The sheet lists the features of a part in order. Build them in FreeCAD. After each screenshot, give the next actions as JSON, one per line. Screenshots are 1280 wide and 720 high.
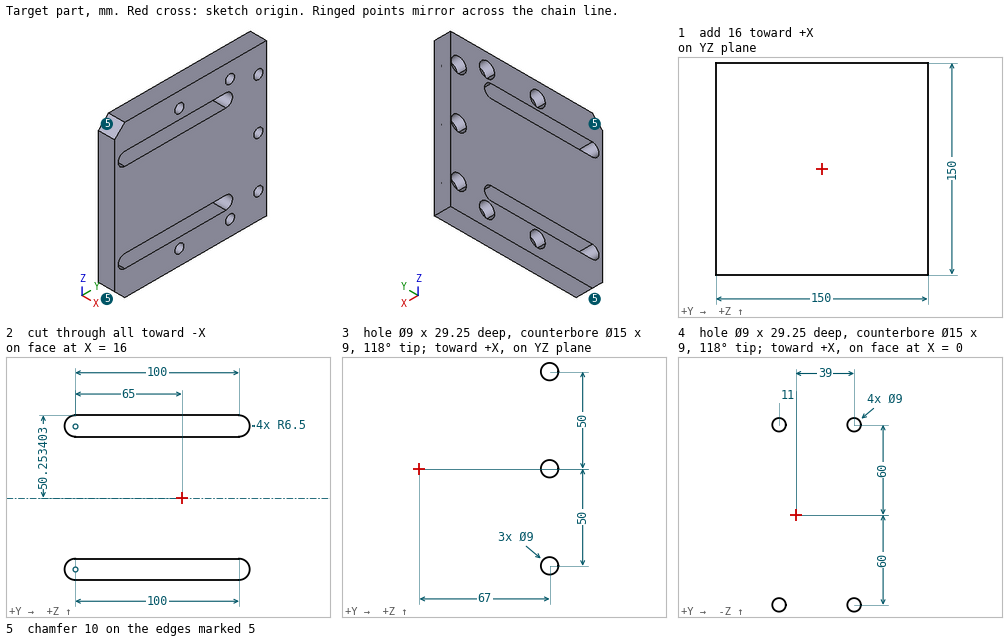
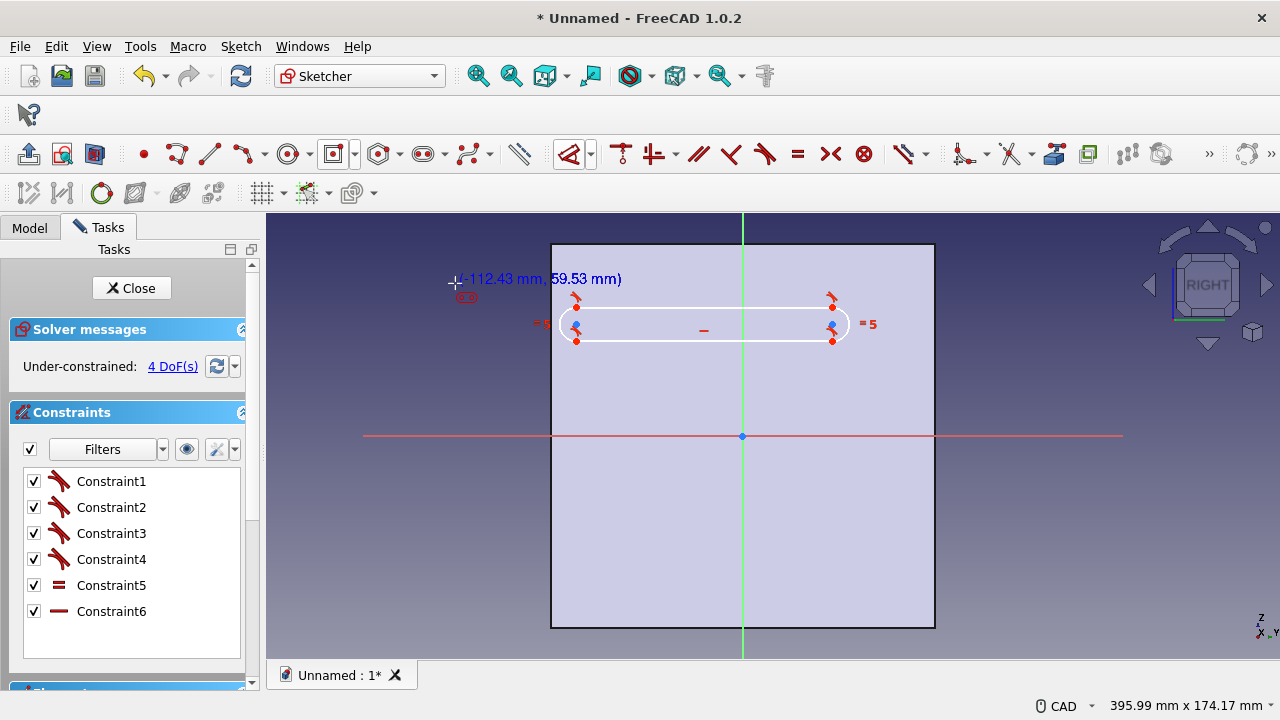
{"action": "scroll", "coordinate": [577, 548], "scroll_direction": "up", "scroll_amount": 2}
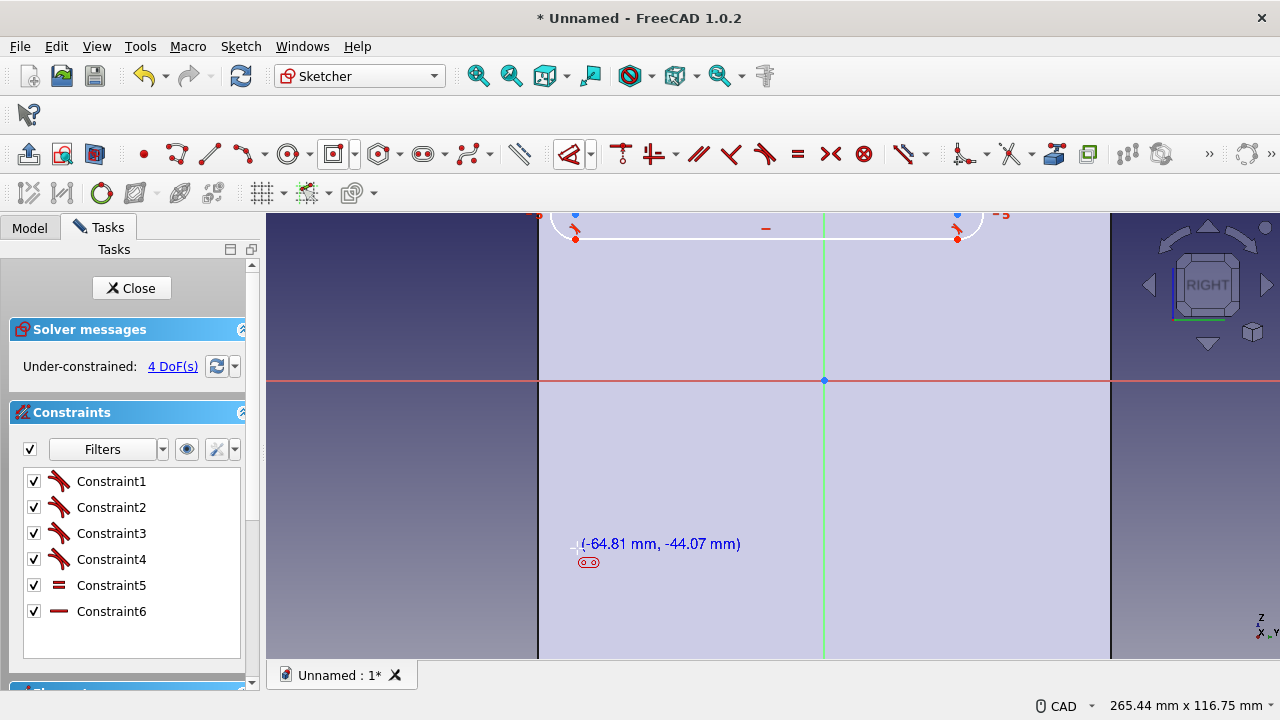
{"action": "left_click", "coordinate": [576, 548]}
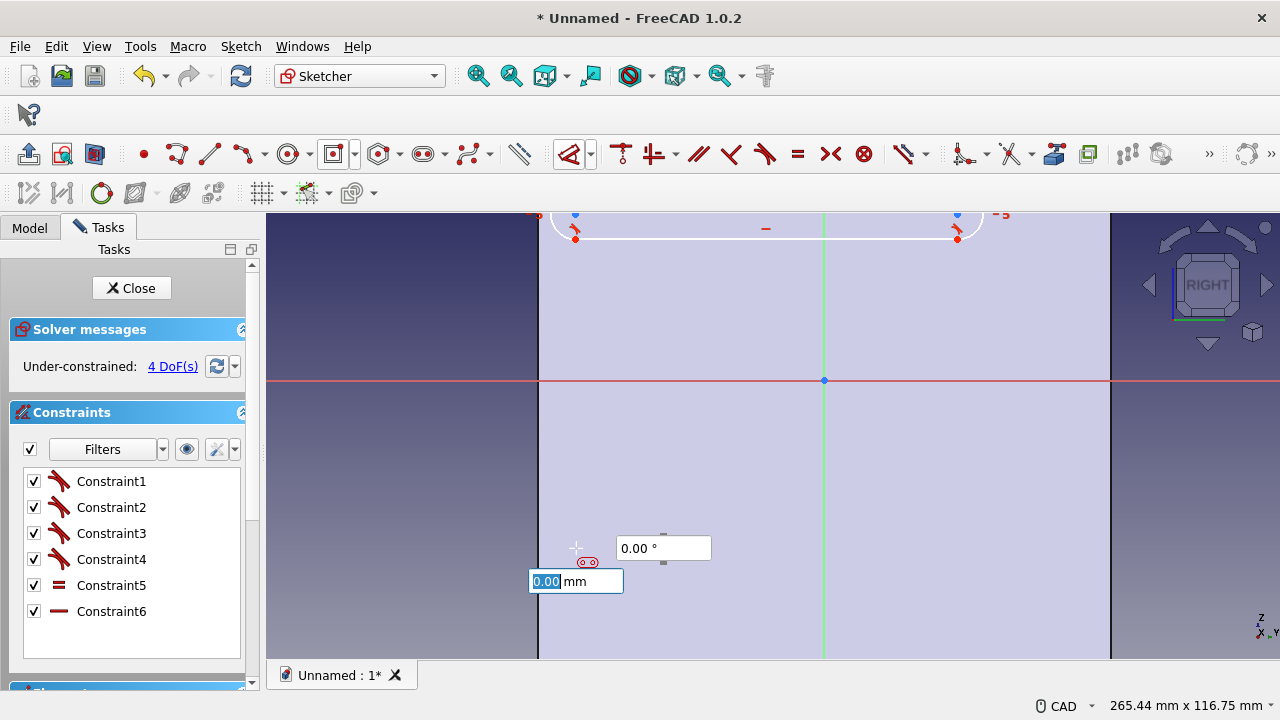
{"action": "left_click", "coordinate": [958, 548]}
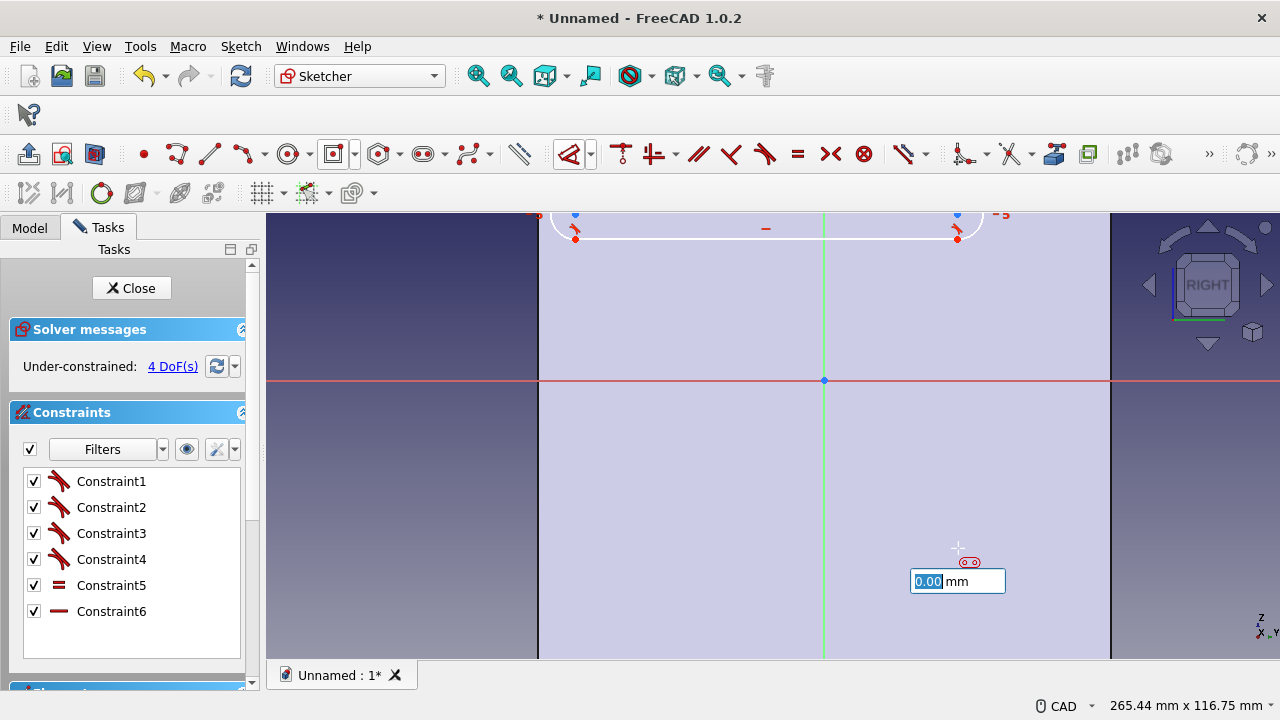
{"action": "left_click", "coordinate": [767, 573]}
{"action": "key", "text": "Escape"}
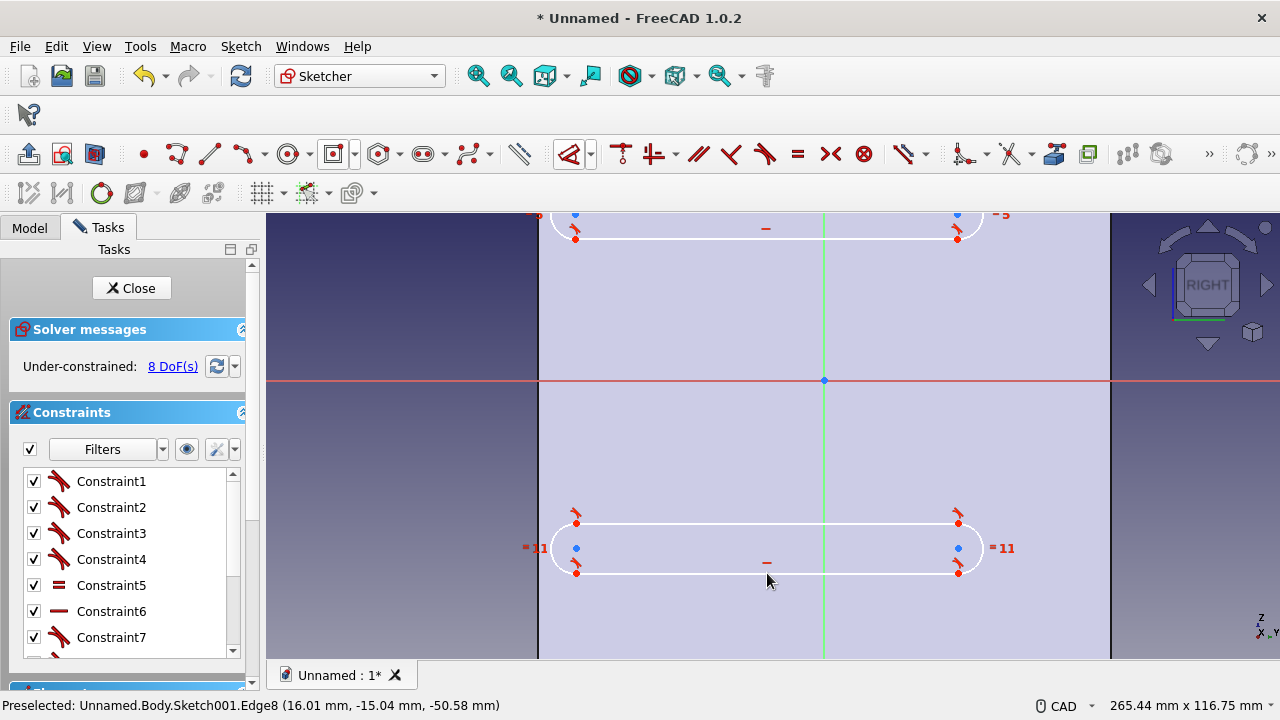
{"action": "scroll", "coordinate": [577, 548], "scroll_direction": "down", "scroll_amount": 2}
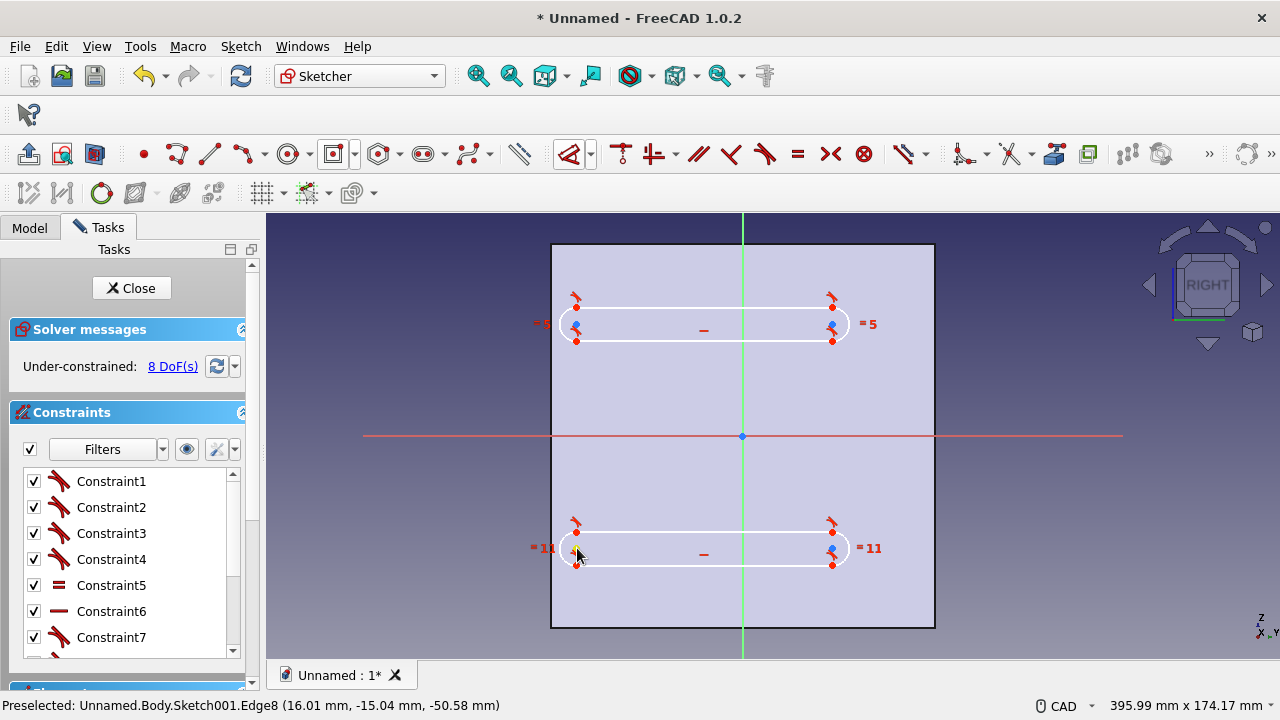
{"action": "left_click", "coordinate": [563, 315]}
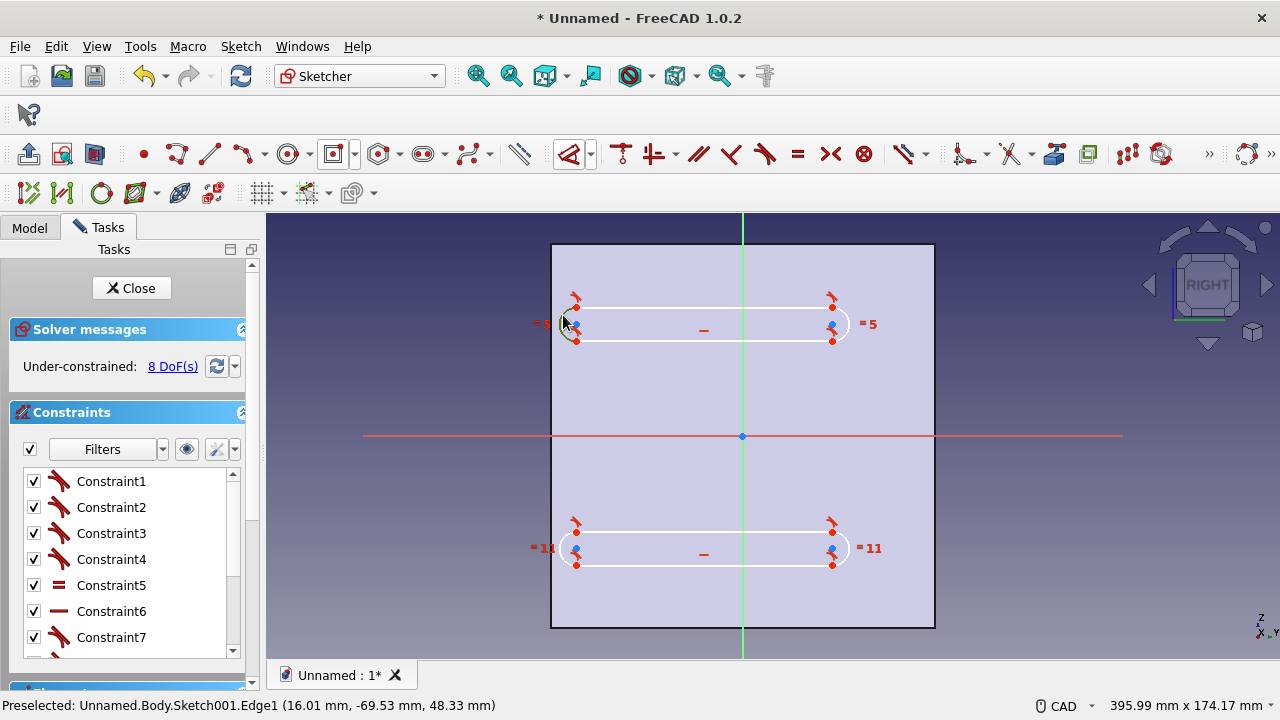
{"action": "left_click", "coordinate": [563, 539]}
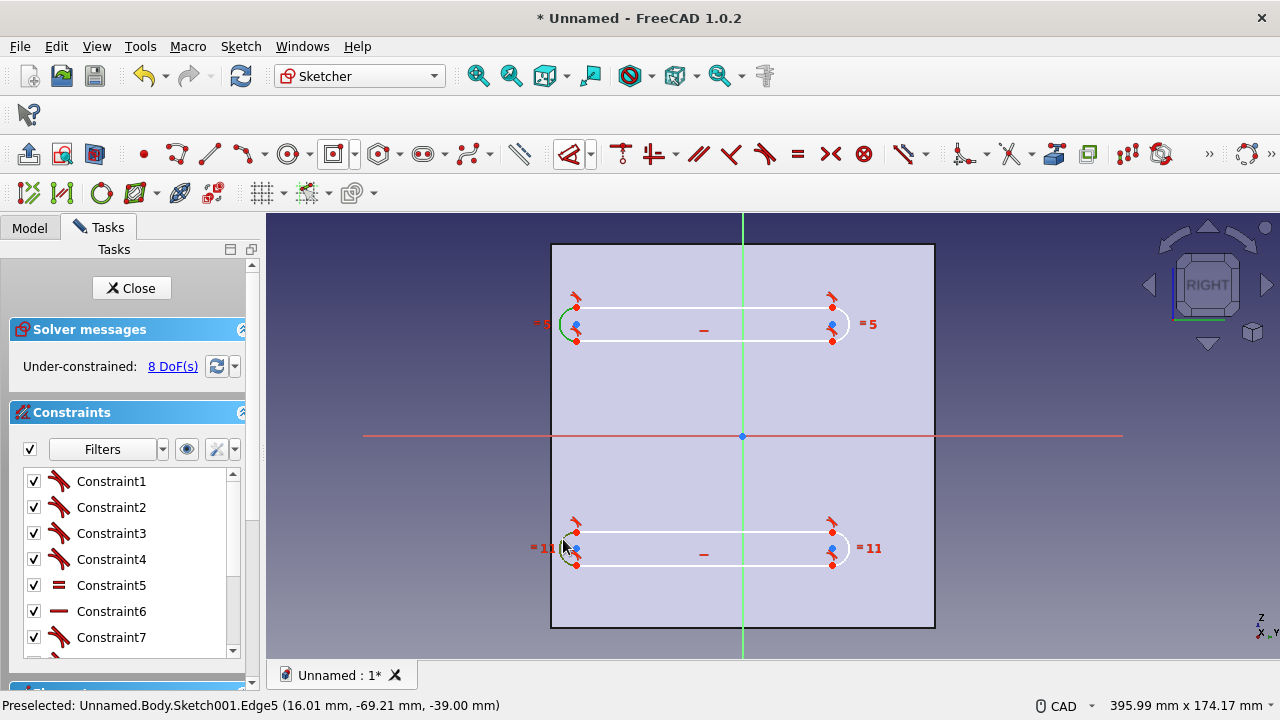
{"action": "key", "text": "e"}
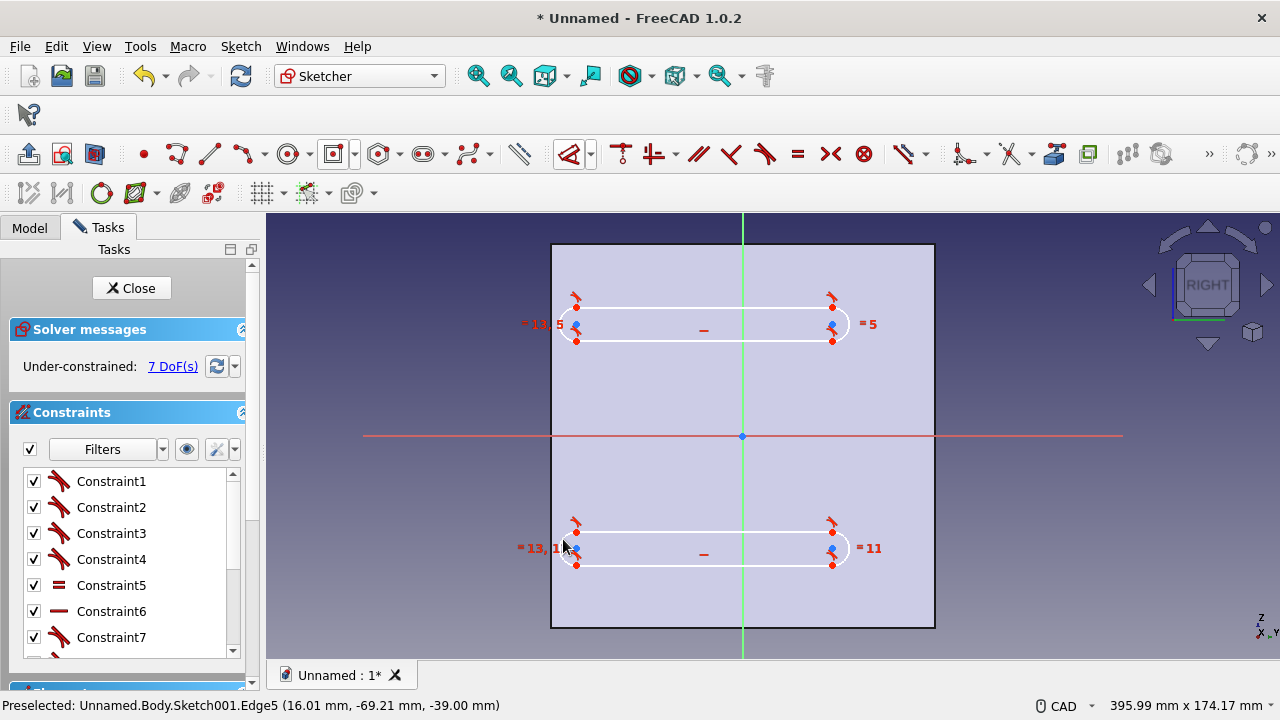
{"action": "left_click", "coordinate": [576, 325]}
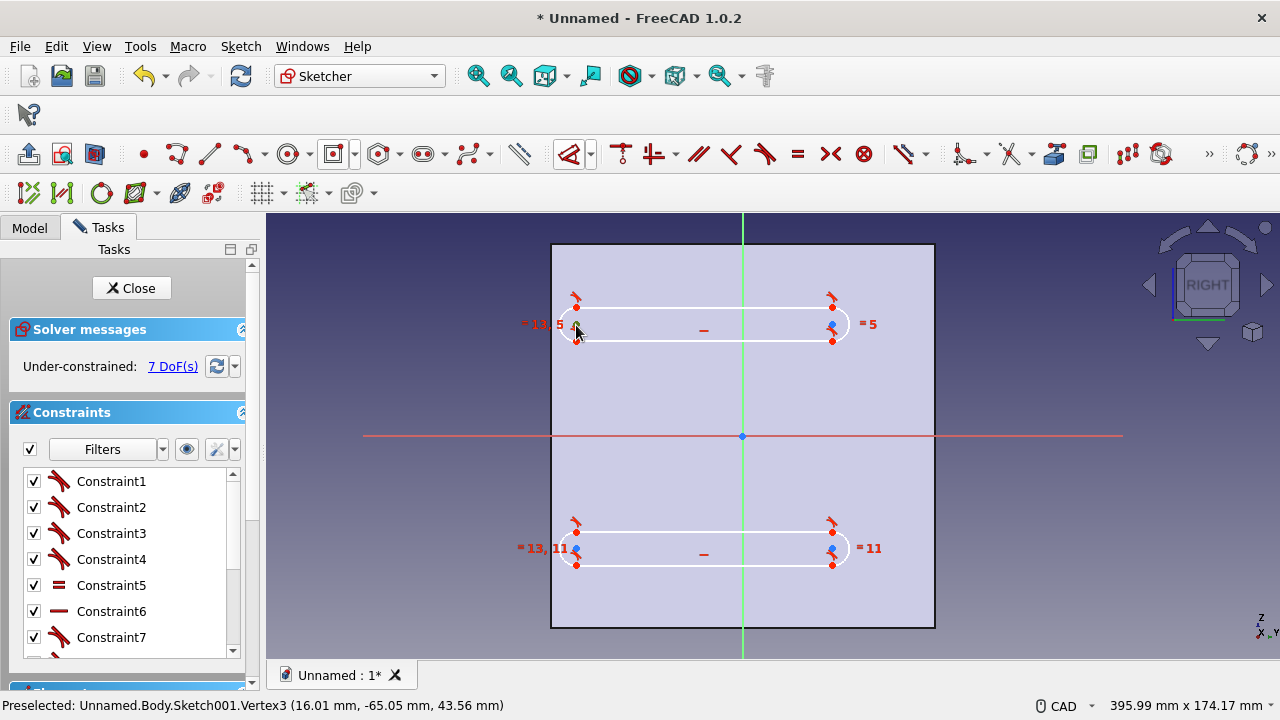
{"action": "left_click", "coordinate": [576, 549]}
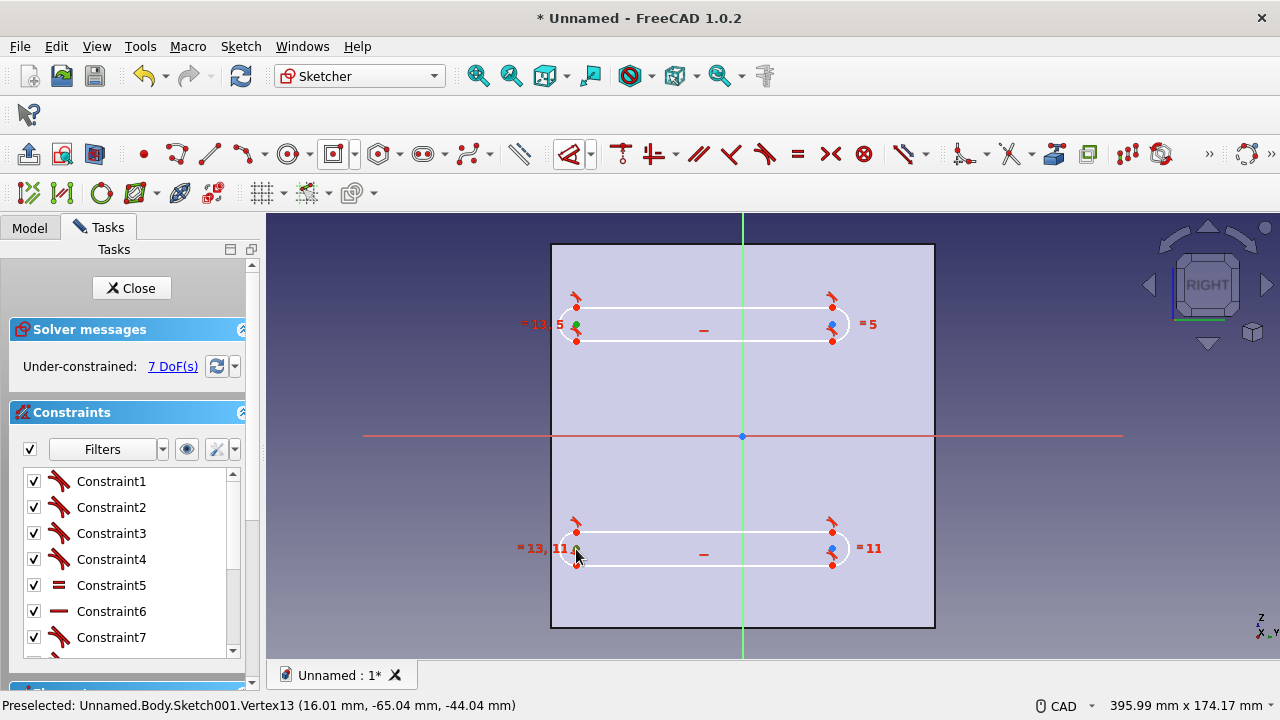
{"action": "left_click", "coordinate": [411, 436]}